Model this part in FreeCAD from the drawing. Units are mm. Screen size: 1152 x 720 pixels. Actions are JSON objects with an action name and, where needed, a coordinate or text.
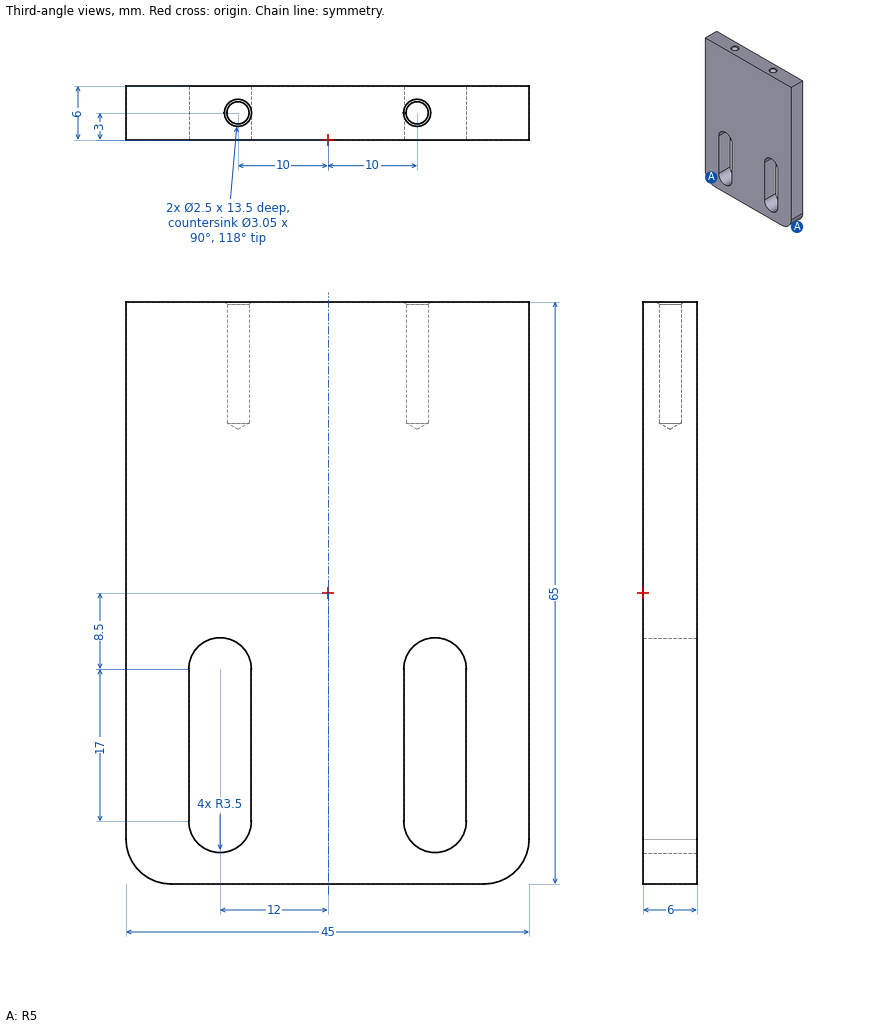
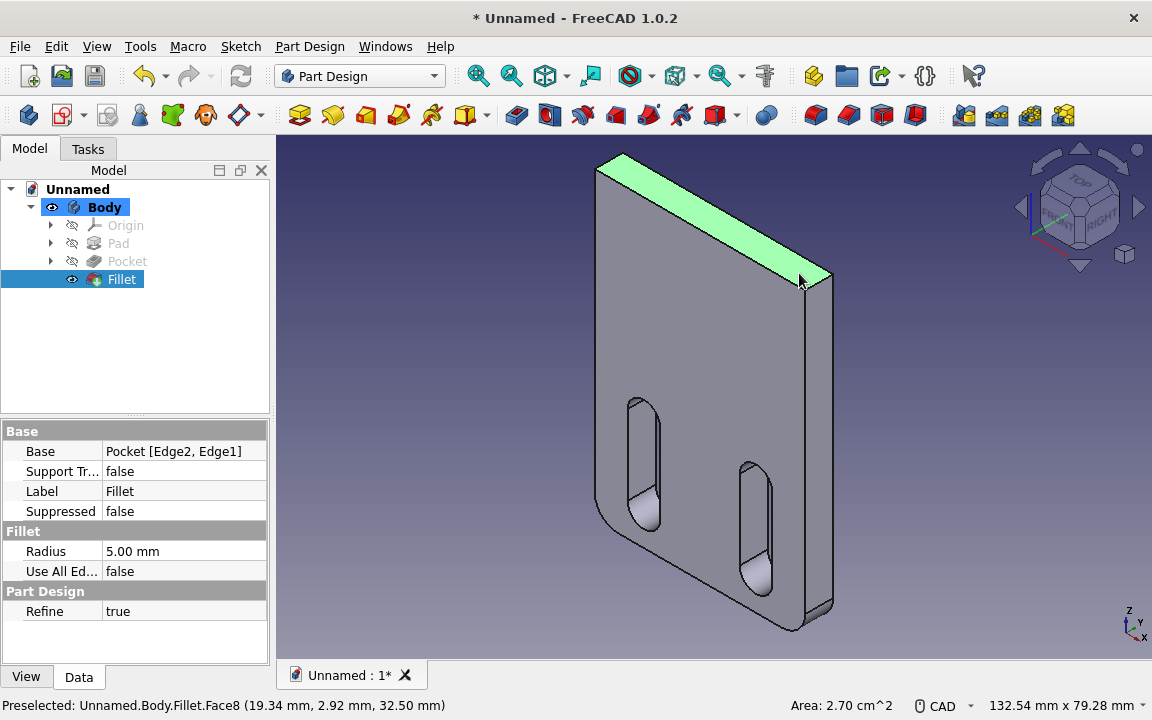
{"action": "left_click", "coordinate": [62, 116]}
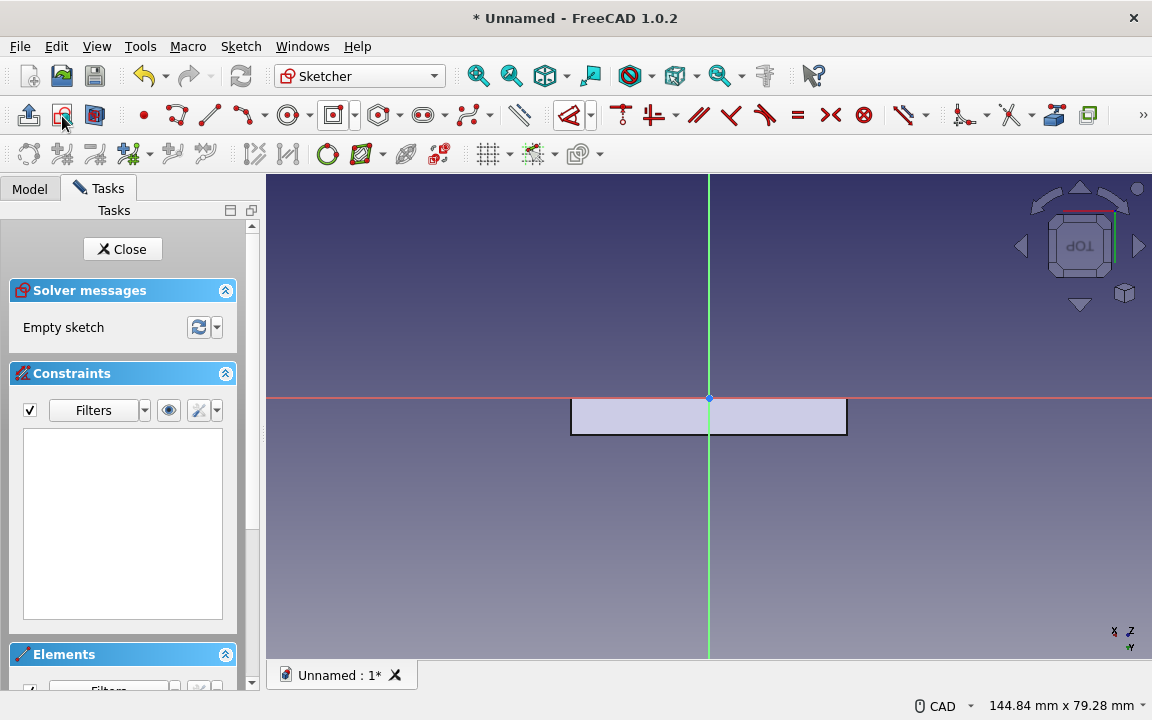
{"action": "scroll", "coordinate": [739, 409], "scroll_direction": "up", "scroll_amount": 6}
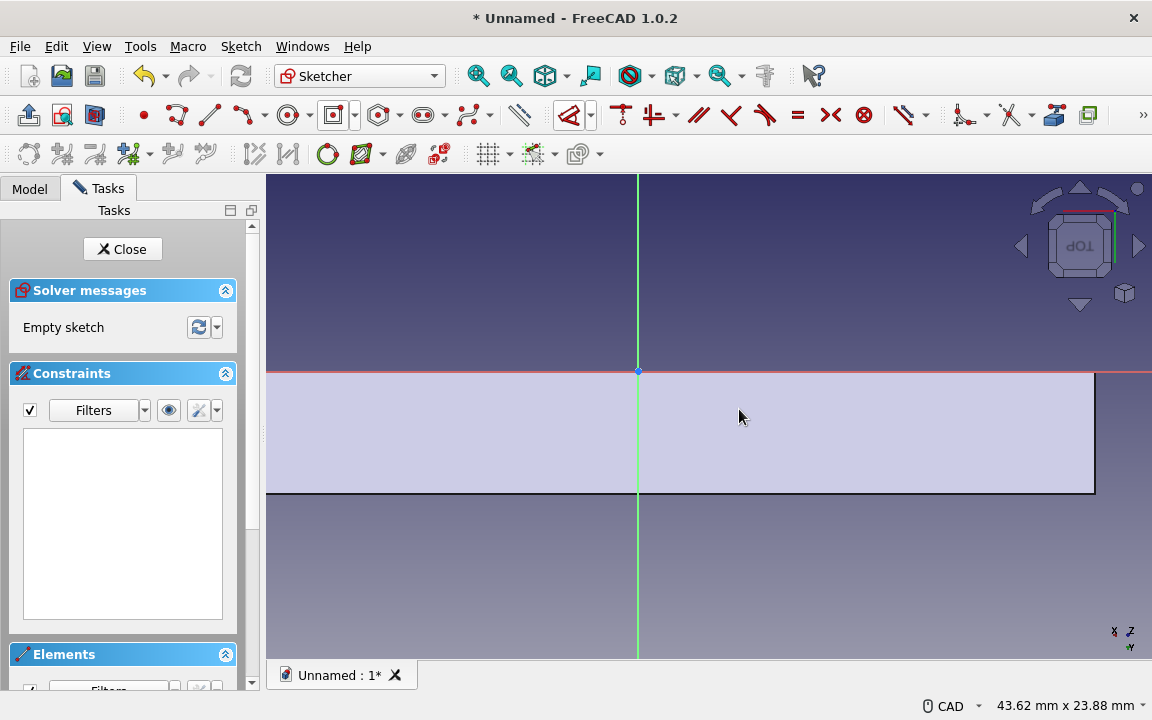
{"action": "left_click", "coordinate": [288, 116]}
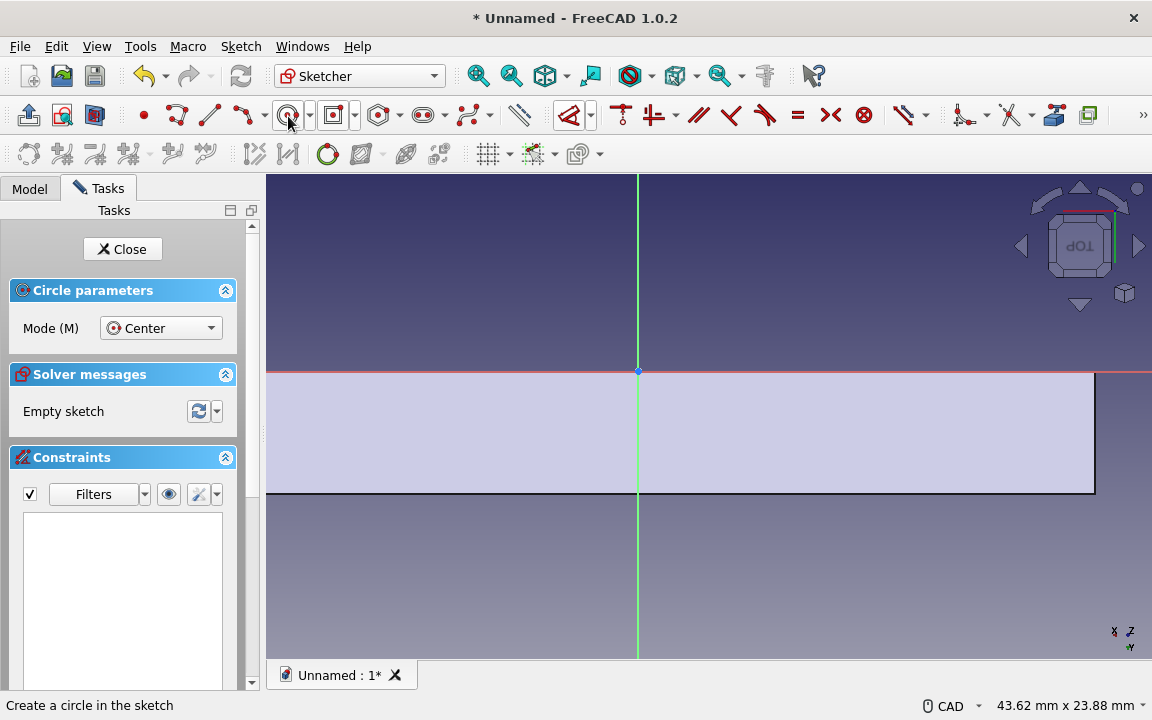
{"action": "left_click", "coordinate": [841, 433]}
{"action": "mouse_move", "coordinate": [859, 415]}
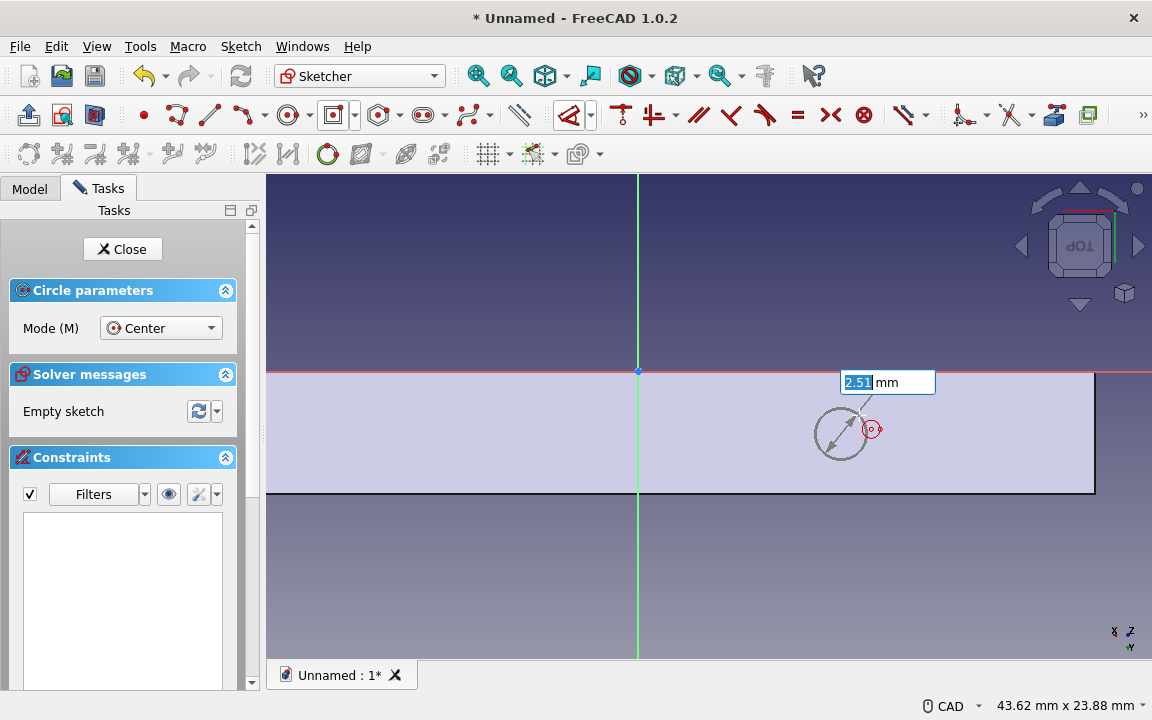
{"action": "type", "text": "2.5"}
{"action": "key", "text": "Return"}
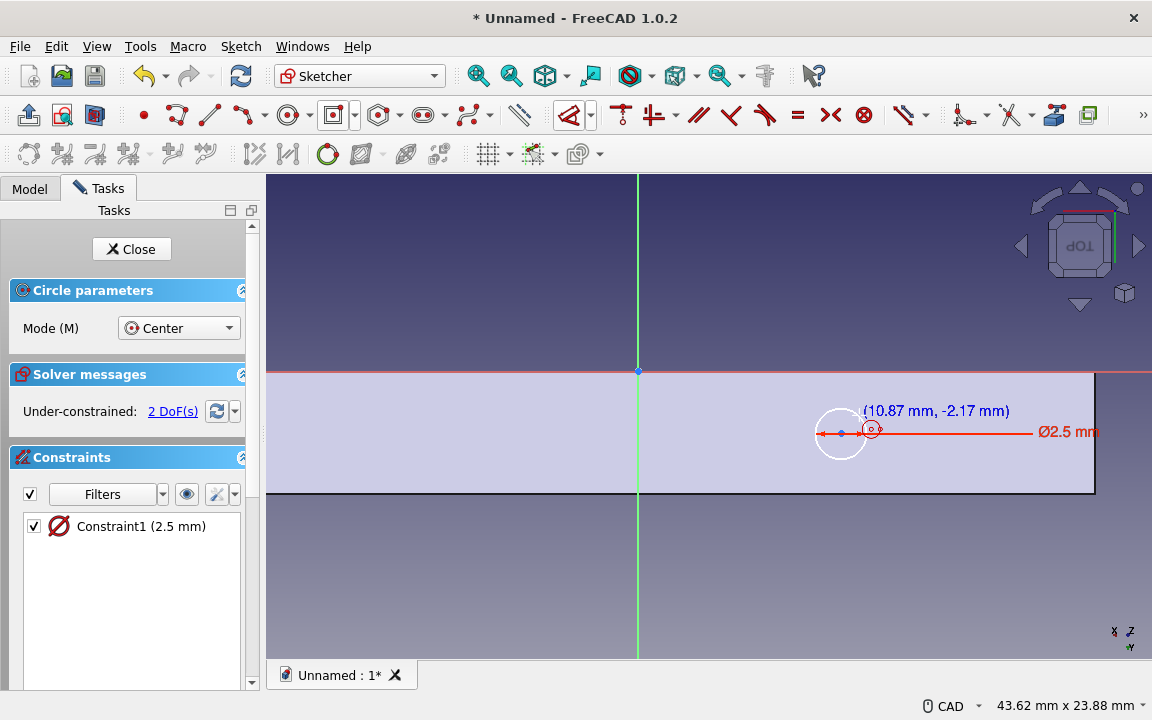
{"action": "left_click", "coordinate": [435, 433]}
{"action": "mouse_move", "coordinate": [453, 415]}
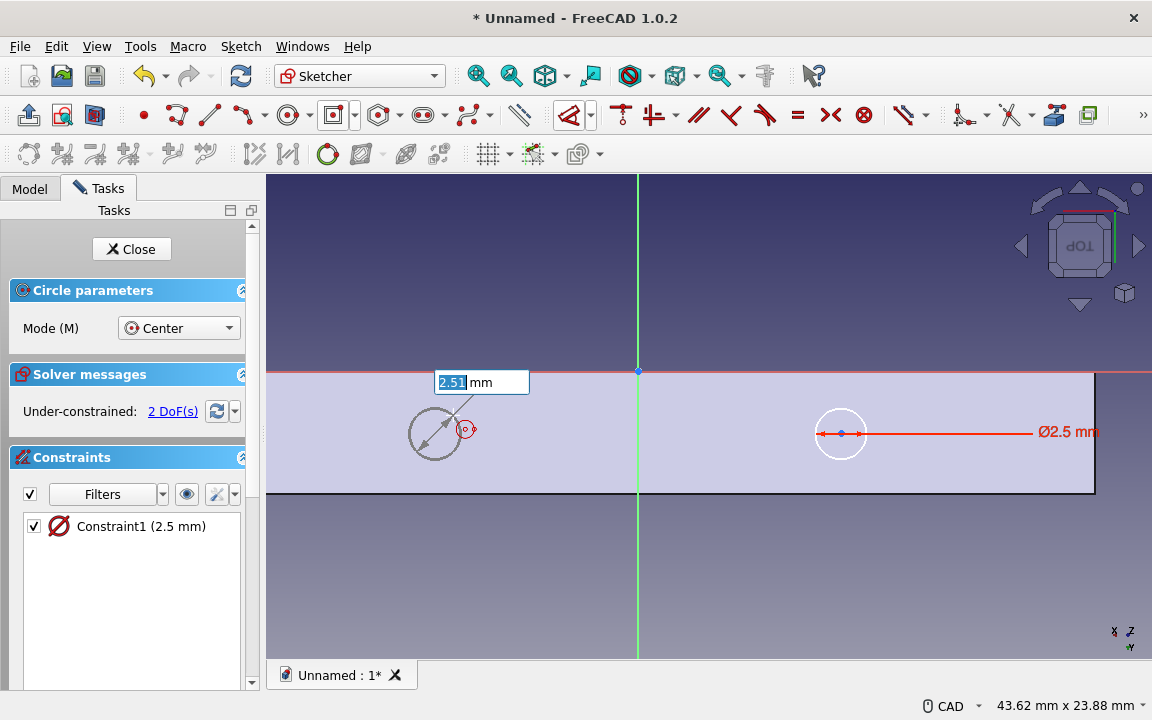
{"action": "type", "text": "2.5"}
{"action": "key", "text": "Return"}
{"action": "key", "text": "Escape"}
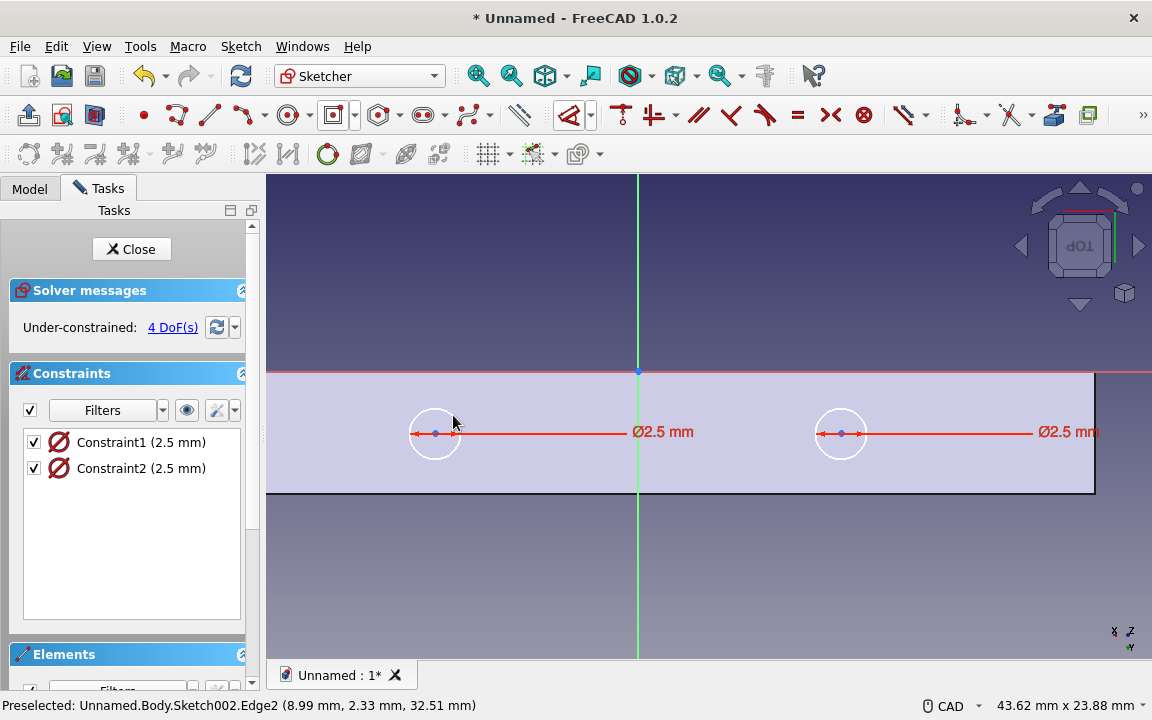
{"action": "left_click", "coordinate": [841, 434]}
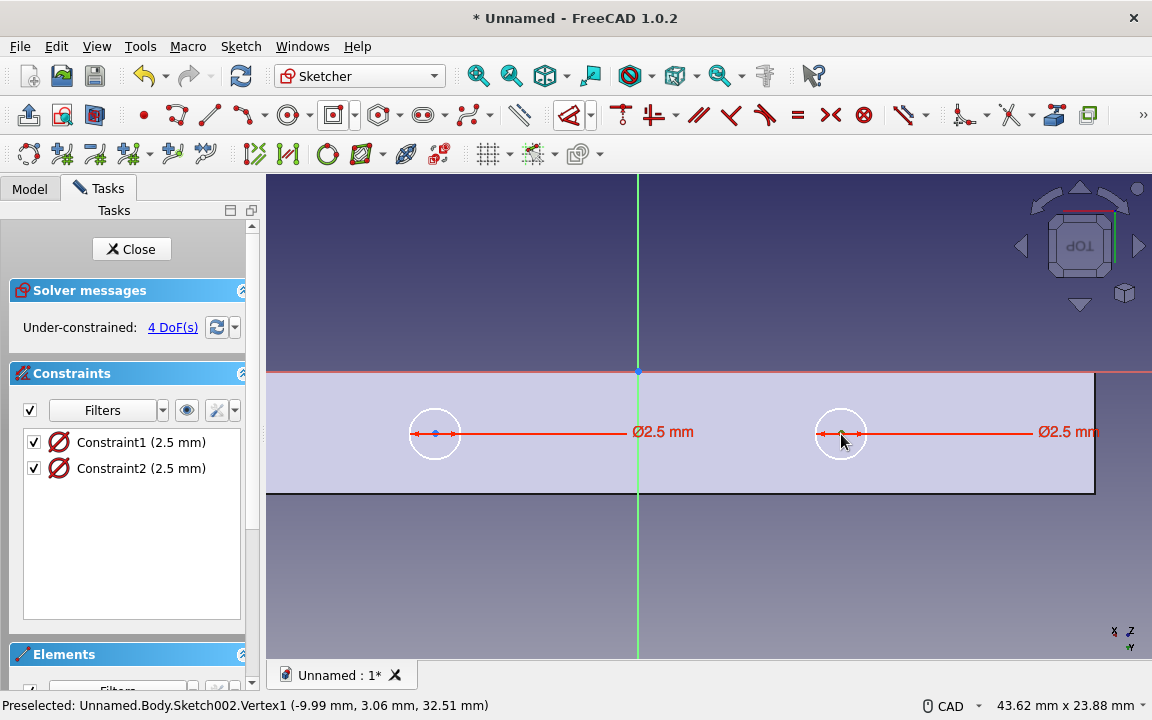
{"action": "left_click", "coordinate": [435, 434]}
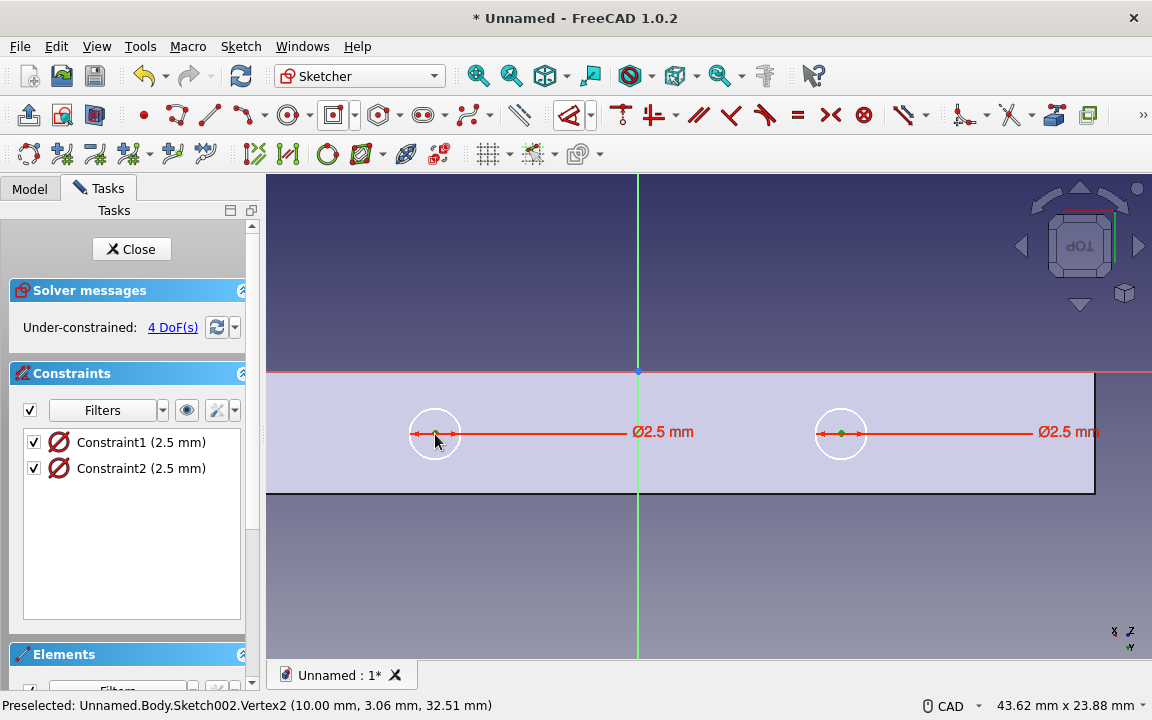
{"action": "key", "text": "h"}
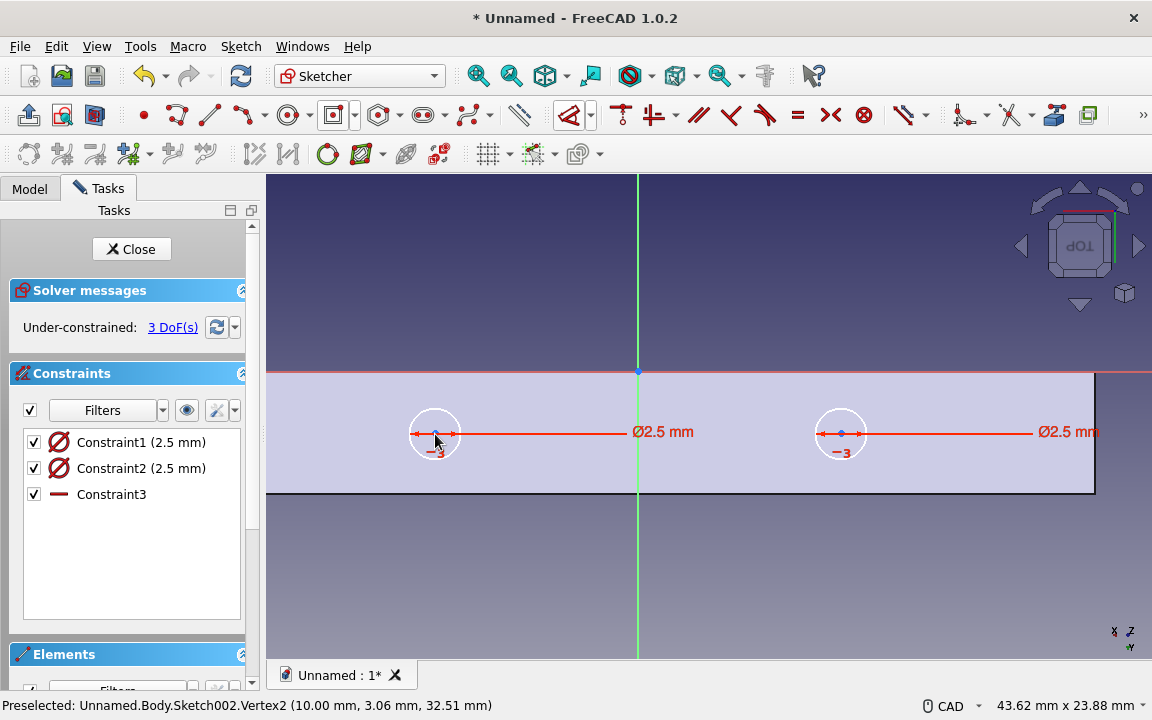
{"action": "left_click", "coordinate": [568, 116]}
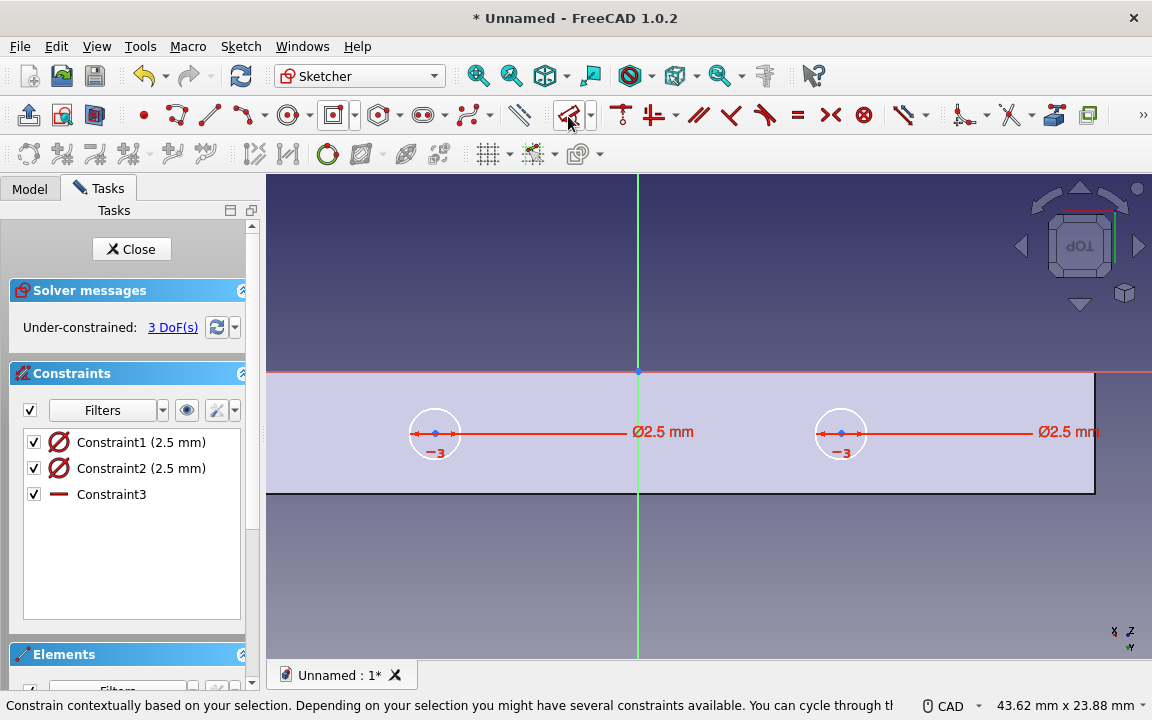
{"action": "left_click", "coordinate": [841, 434]}
{"action": "left_click", "coordinate": [875, 403]}